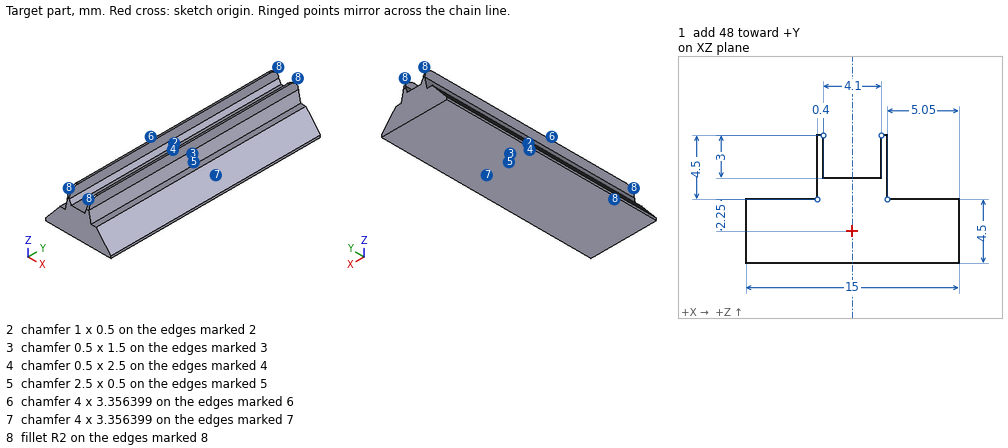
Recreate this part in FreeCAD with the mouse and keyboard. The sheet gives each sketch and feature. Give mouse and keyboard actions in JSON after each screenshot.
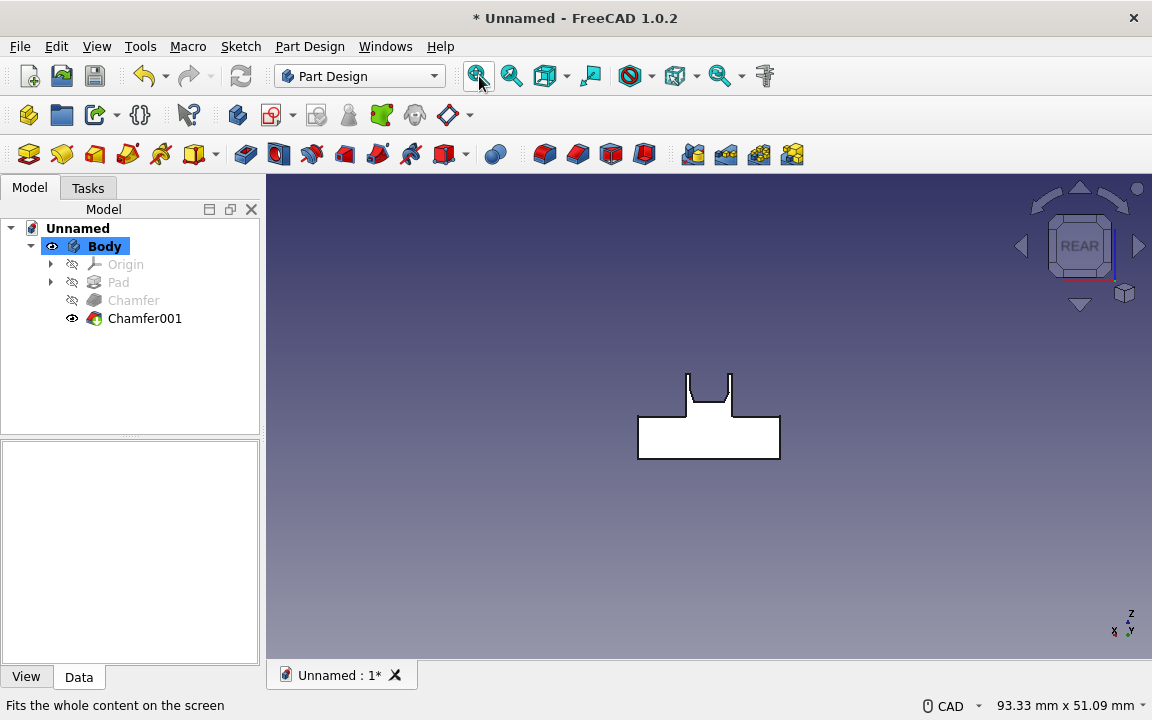
{"action": "key", "text": "6"}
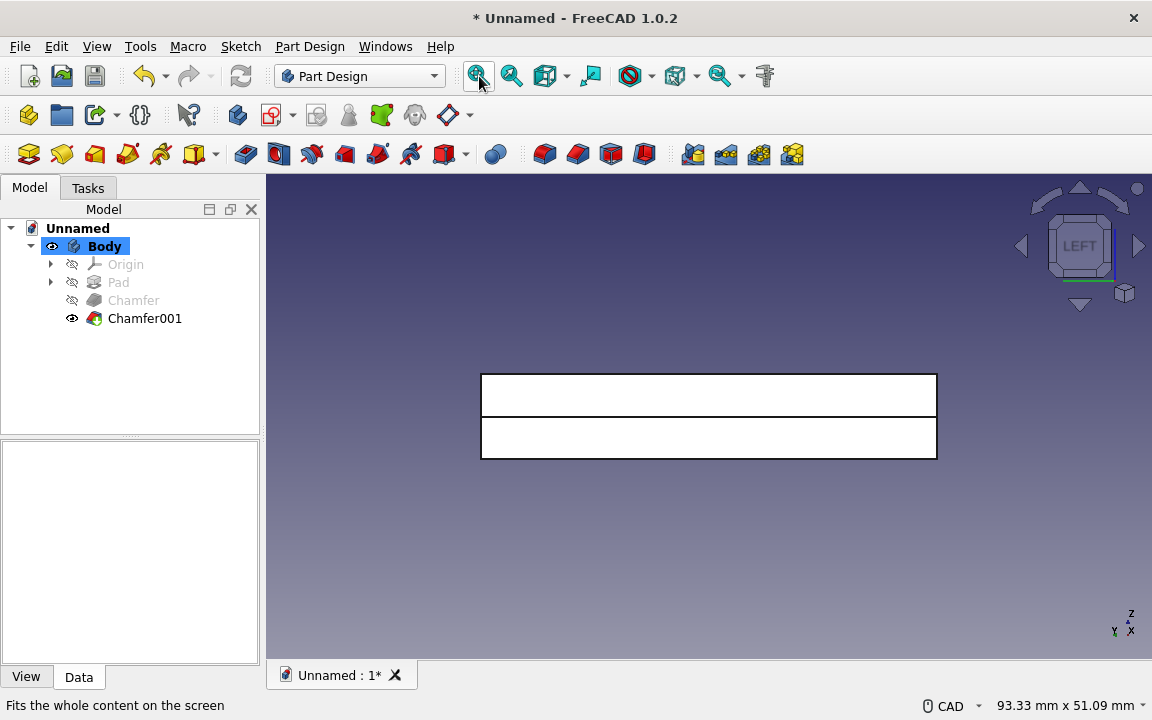
{"action": "key", "text": "v 3"}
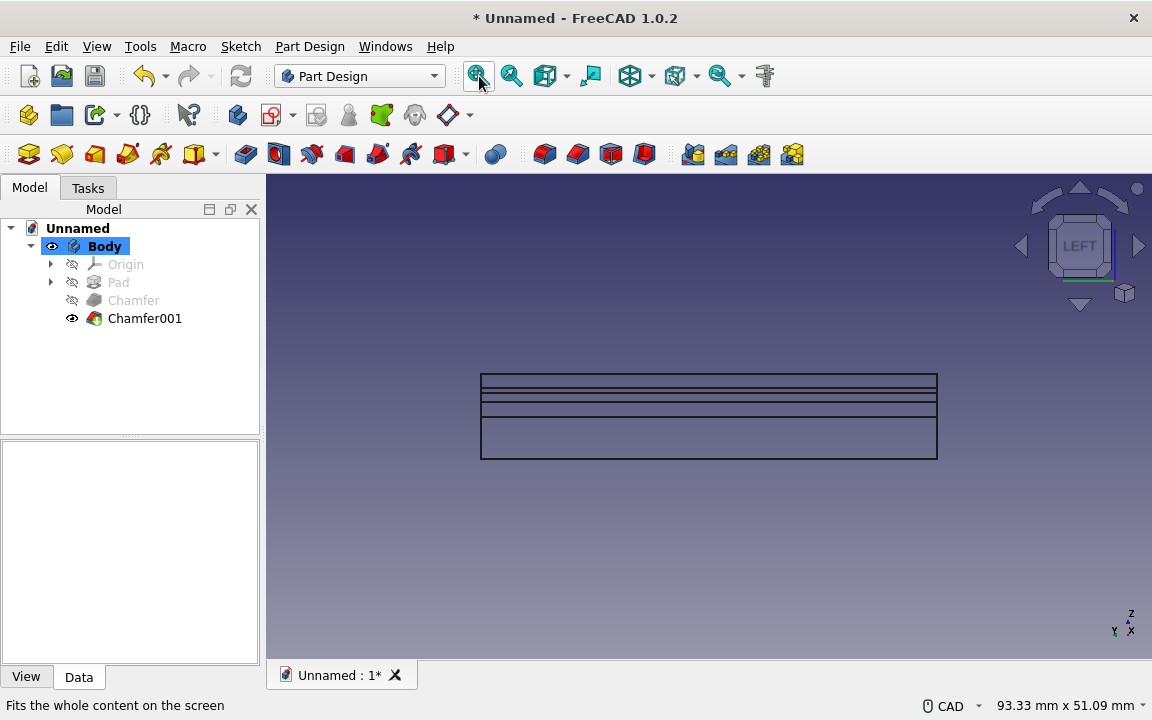
{"action": "key", "text": "0"}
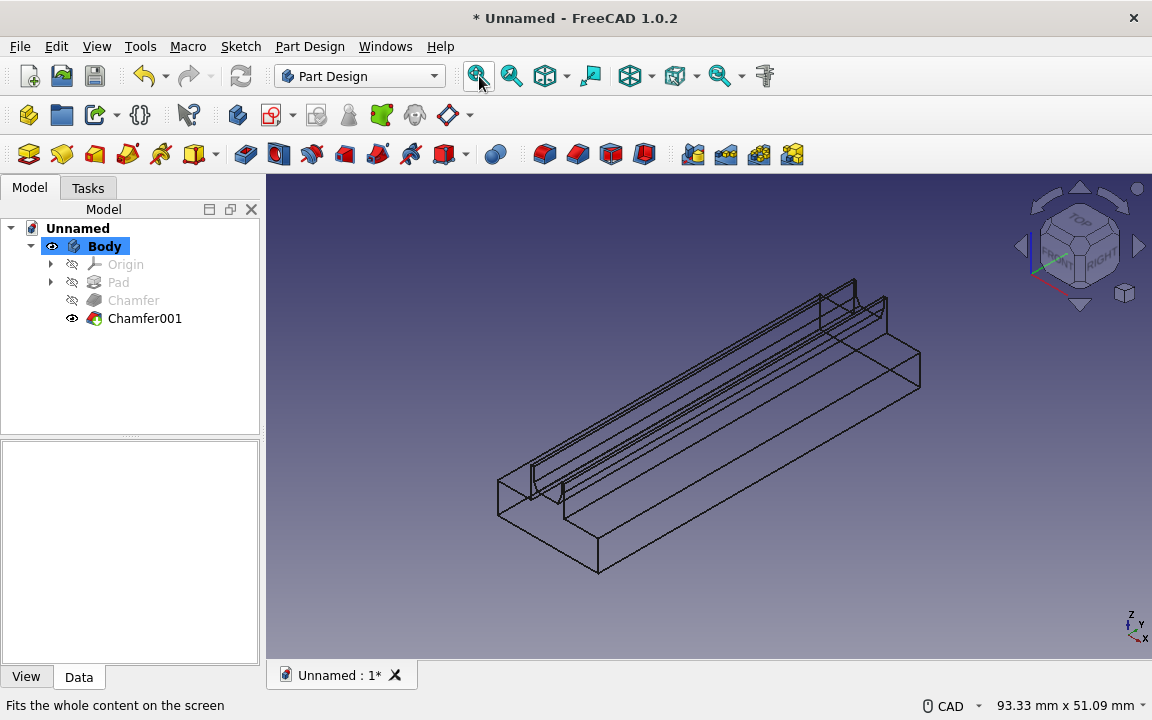
{"action": "key", "text": "2"}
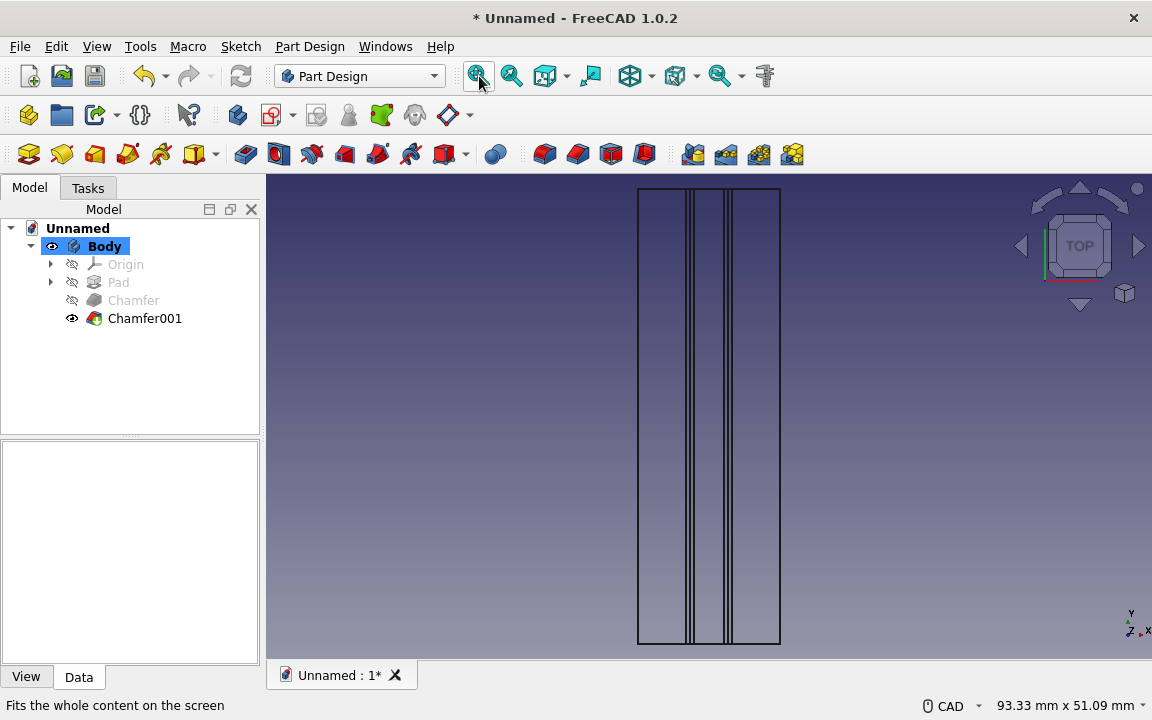
{"action": "key", "text": "1"}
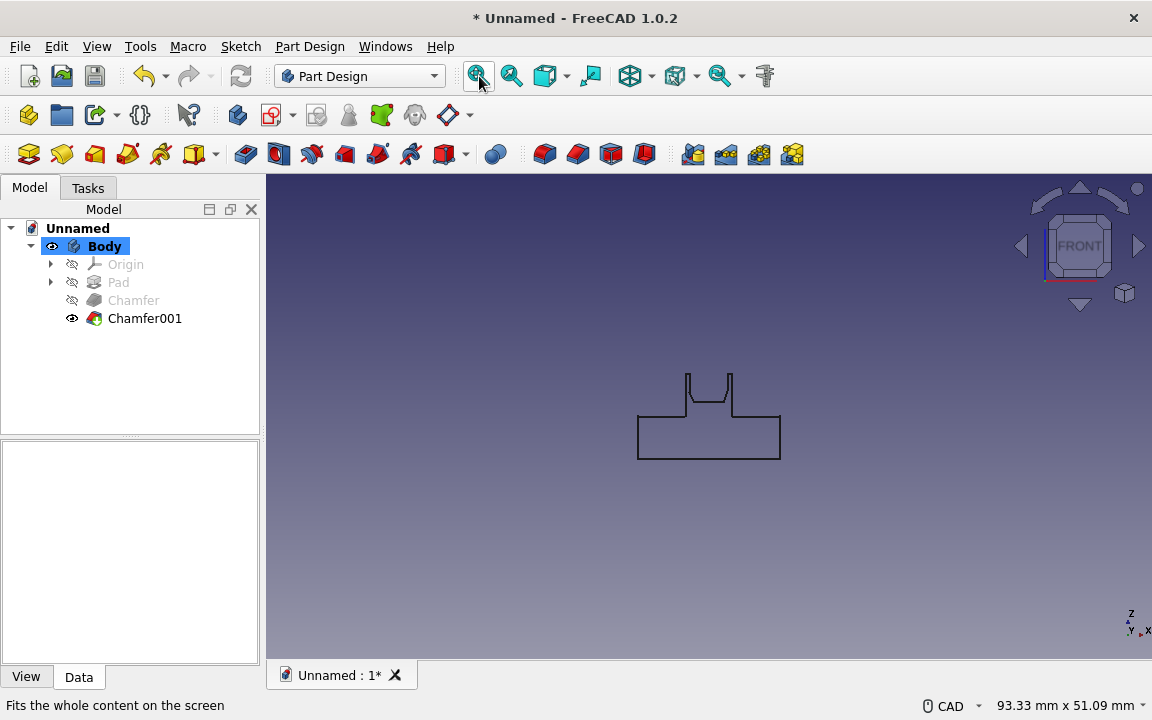
{"action": "left_click", "coordinate": [479, 76]}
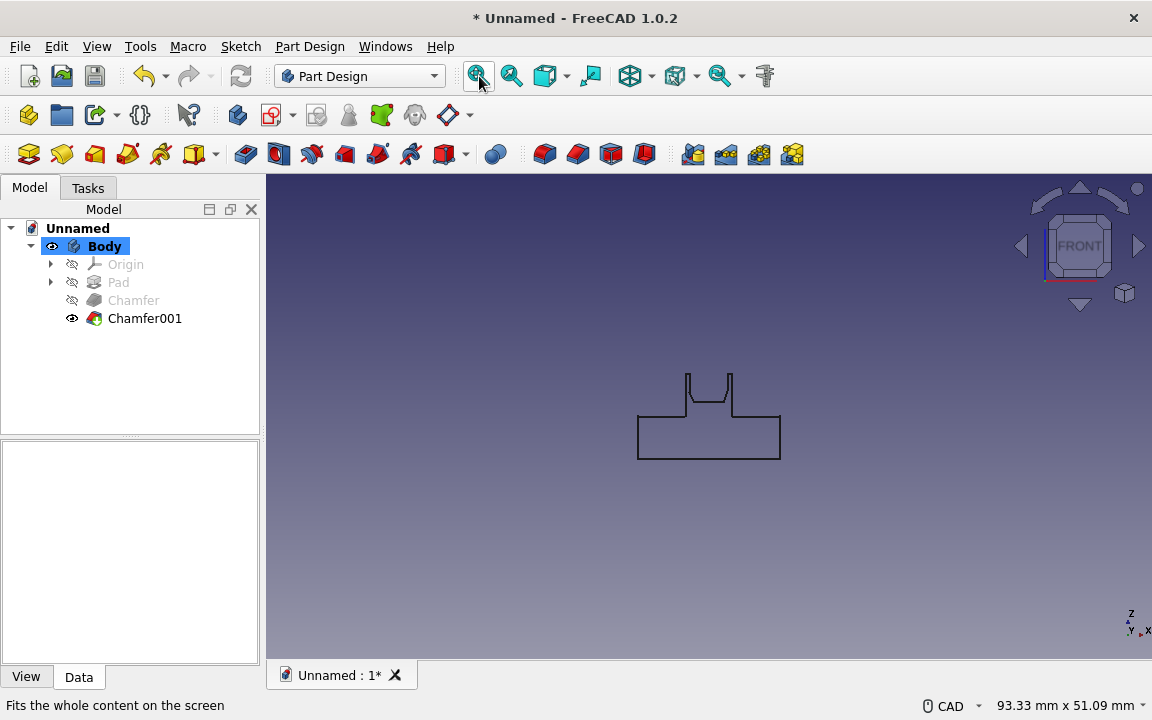
{"action": "key", "text": "3"}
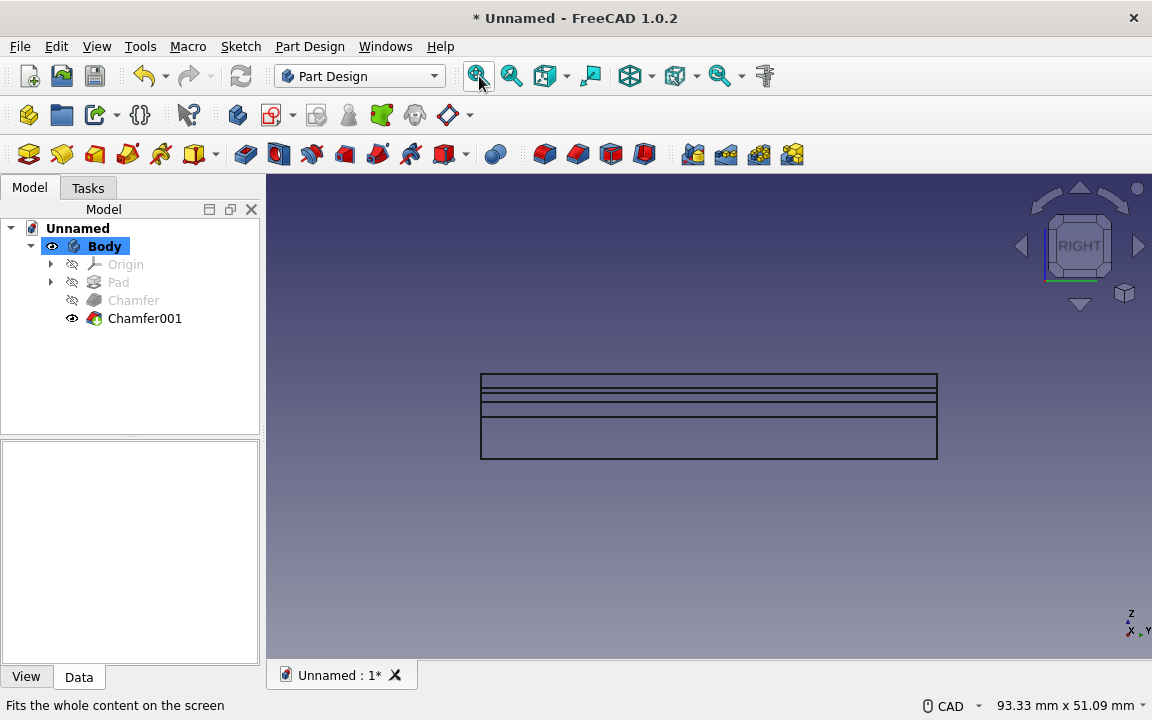
{"action": "key", "text": "5"}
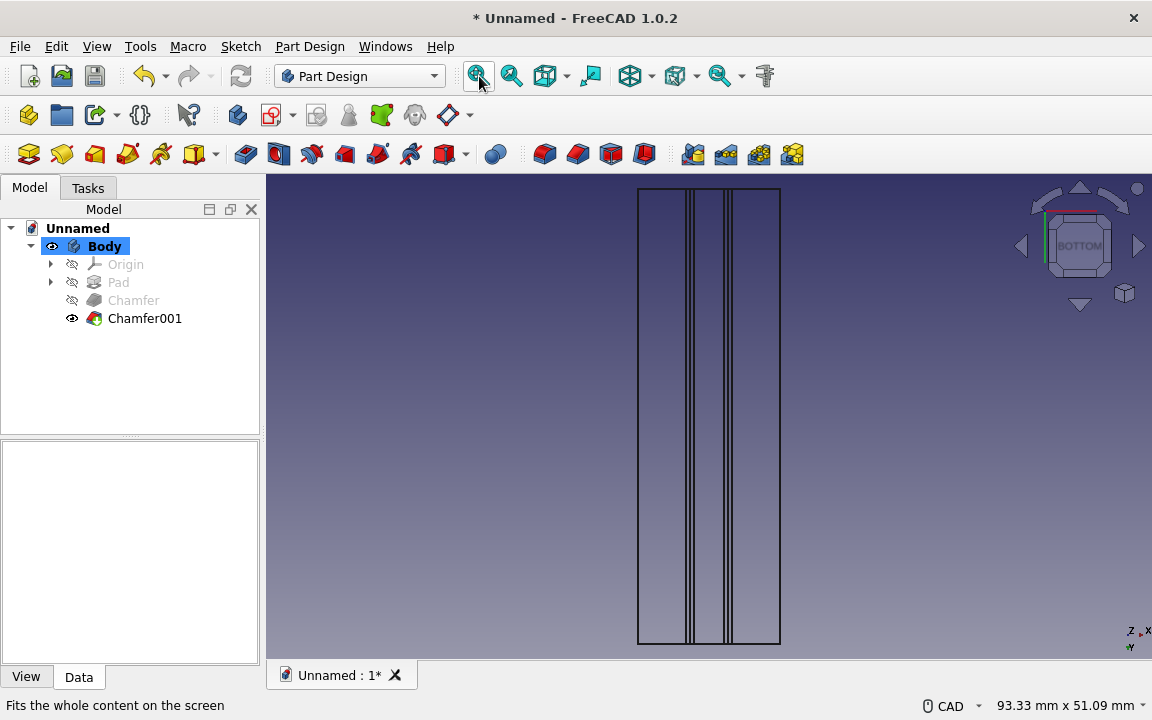
{"action": "left_click", "coordinate": [686, 415]}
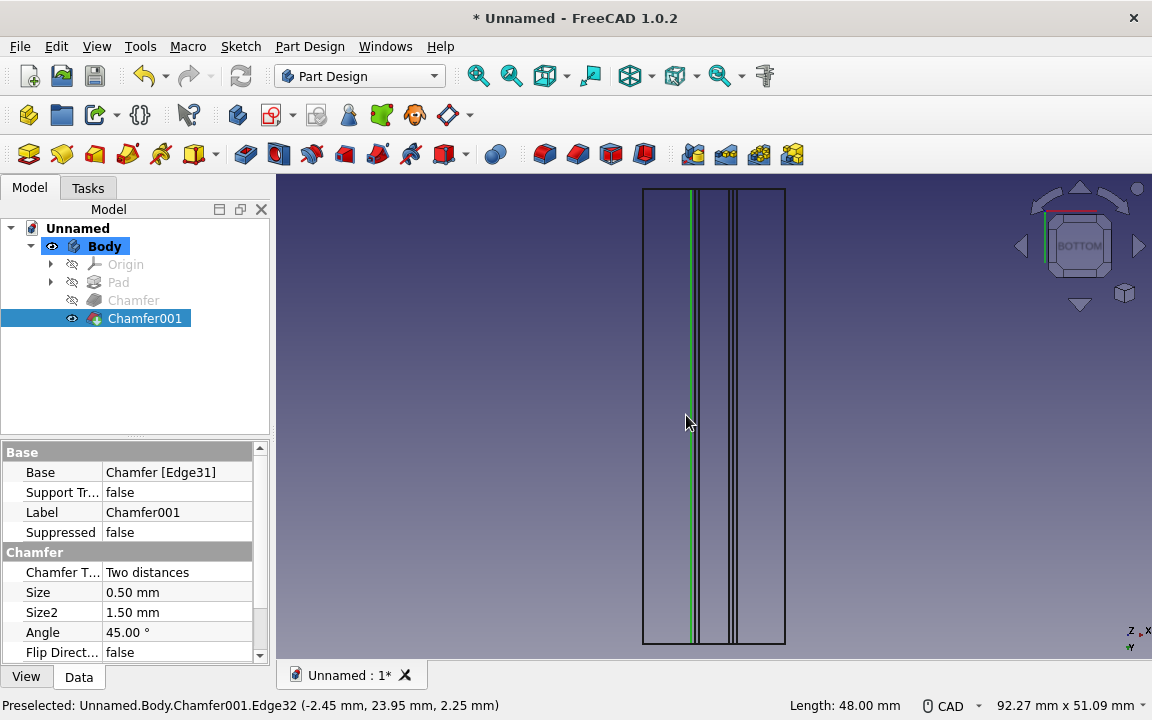
{"action": "key", "text": "v 1"}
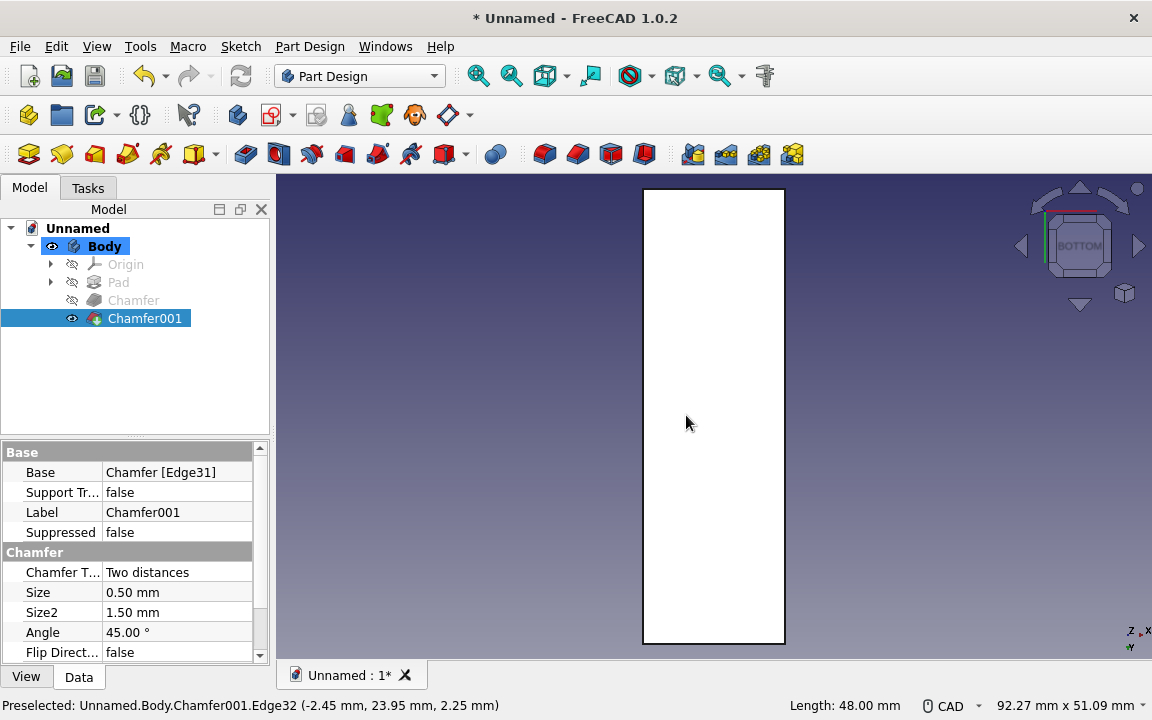
{"action": "left_click", "coordinate": [578, 154]}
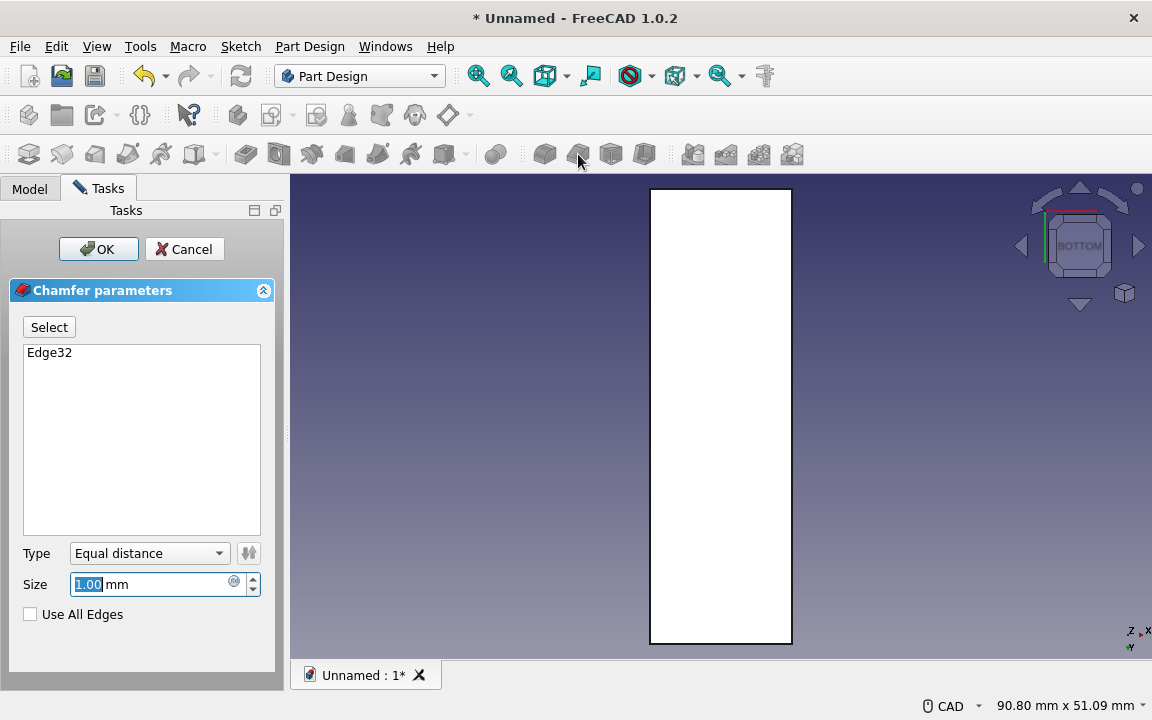
{"action": "type", "text": "0.5"}
{"action": "key", "text": "Tab"}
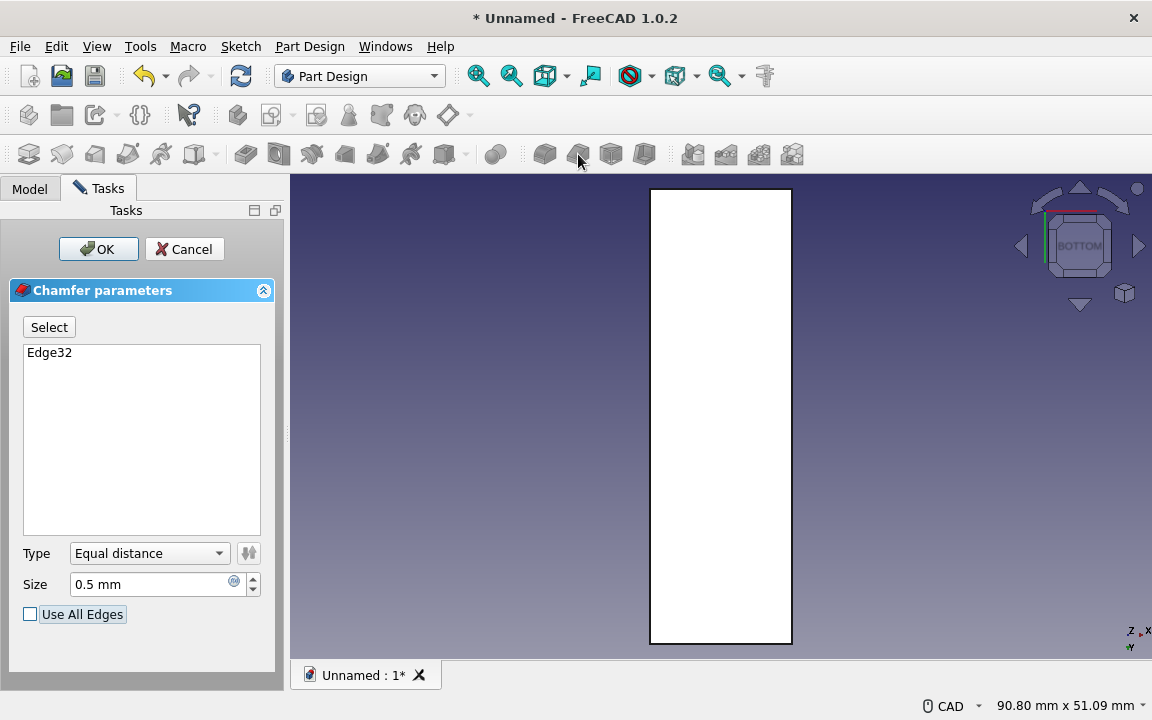
{"action": "left_click", "coordinate": [150, 554]}